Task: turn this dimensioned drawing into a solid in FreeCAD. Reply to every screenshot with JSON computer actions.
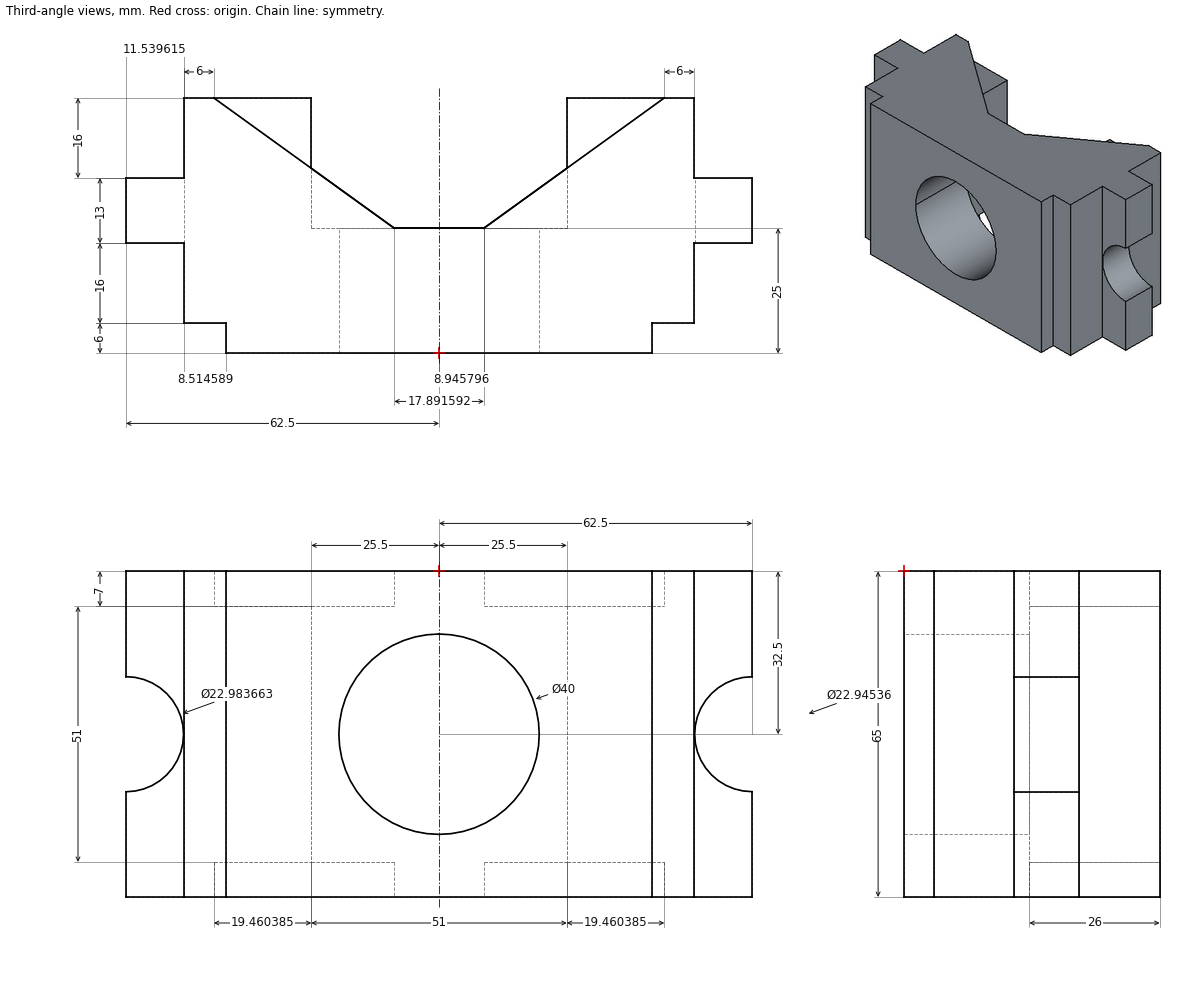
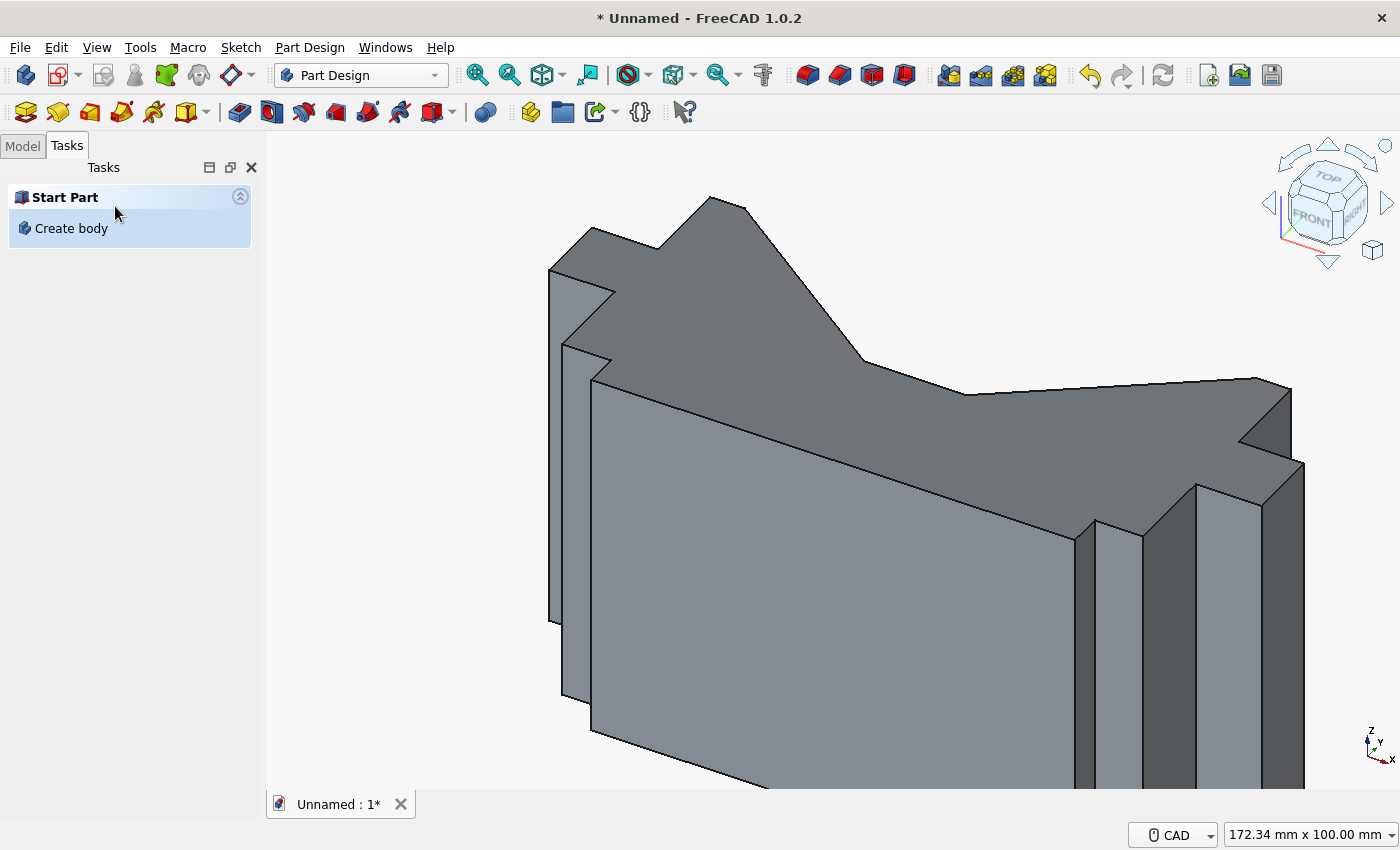
{"action": "left_click", "coordinate": [478, 76]}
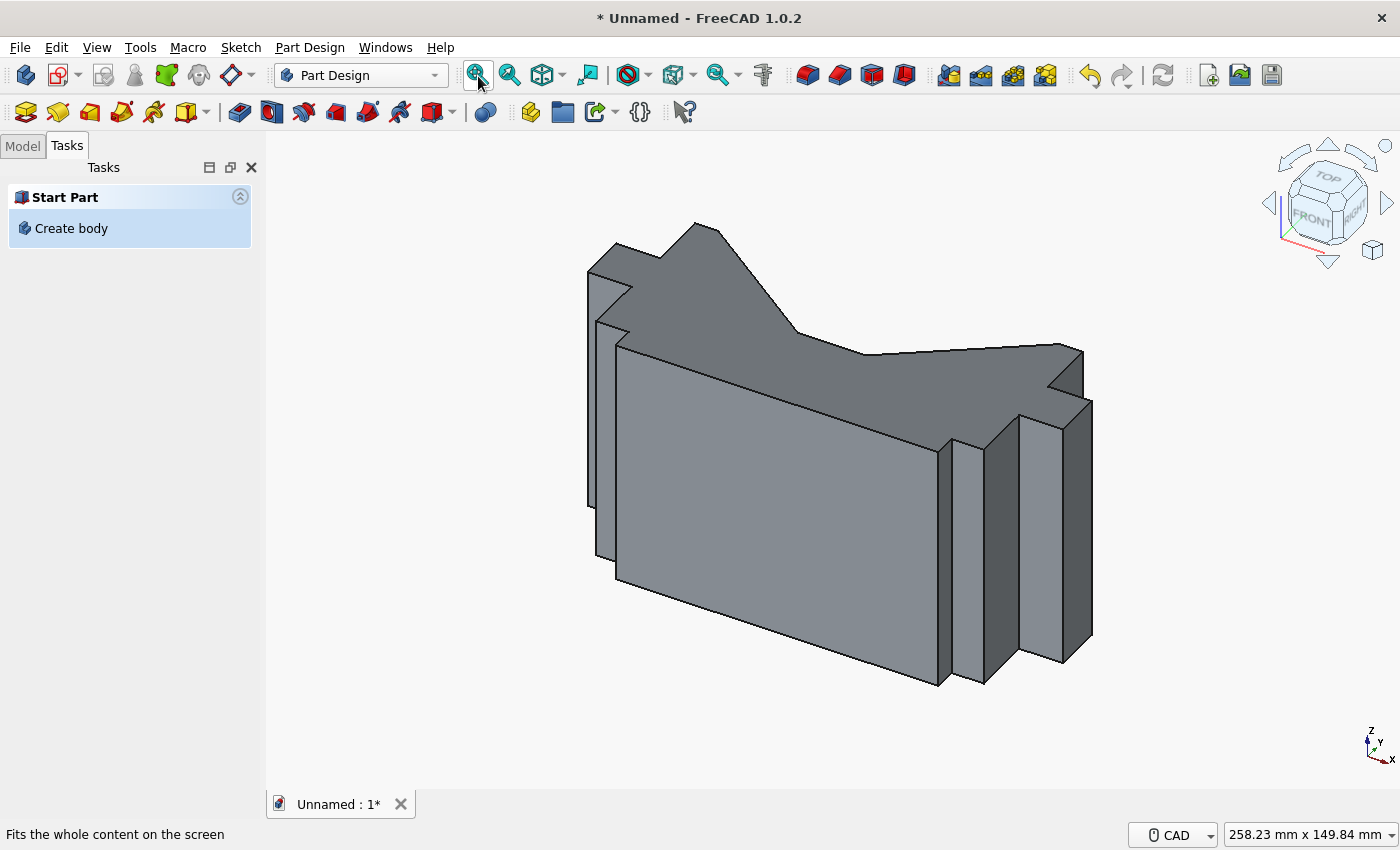
{"action": "key", "text": "4"}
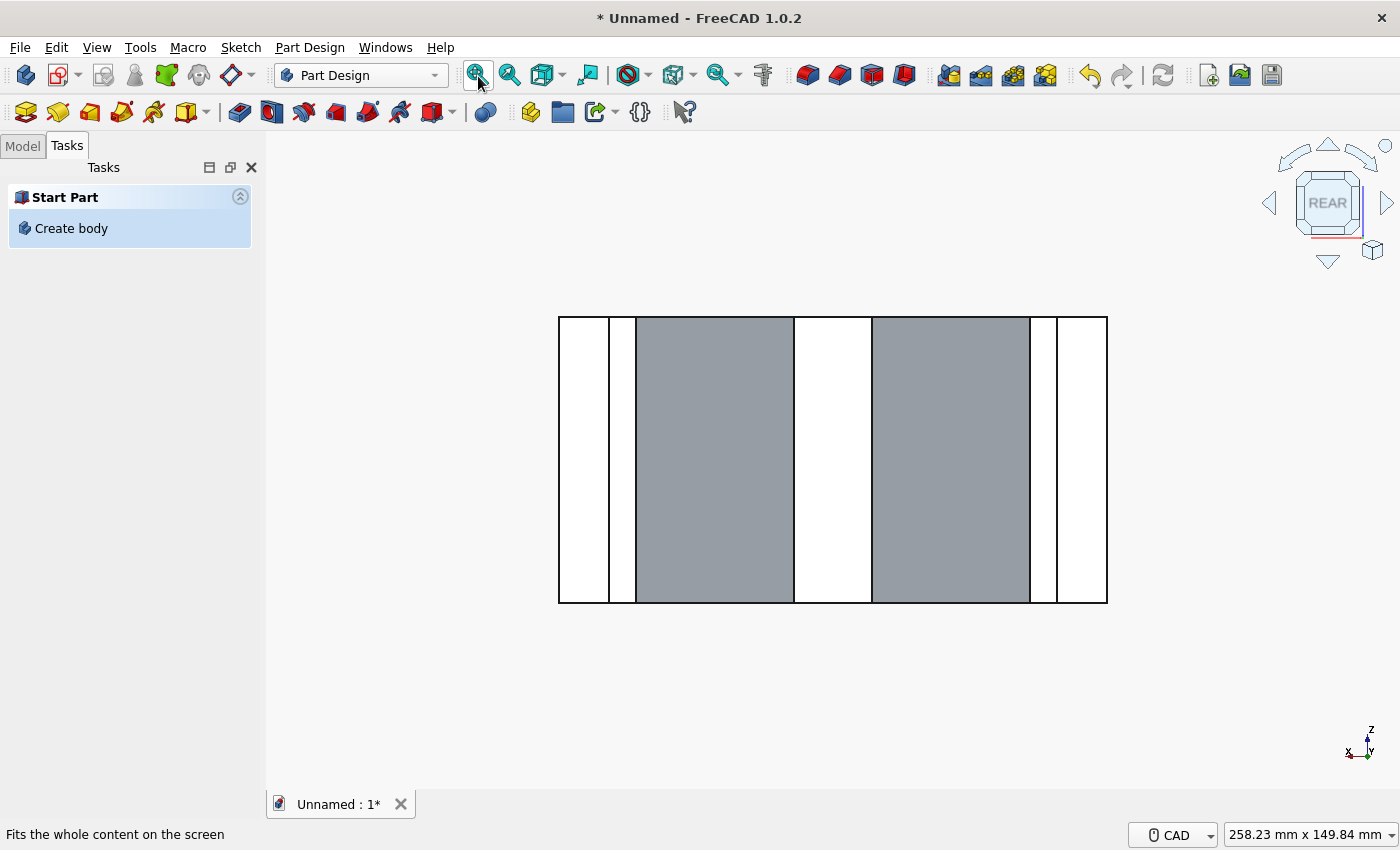
{"action": "left_click", "coordinate": [833, 377]}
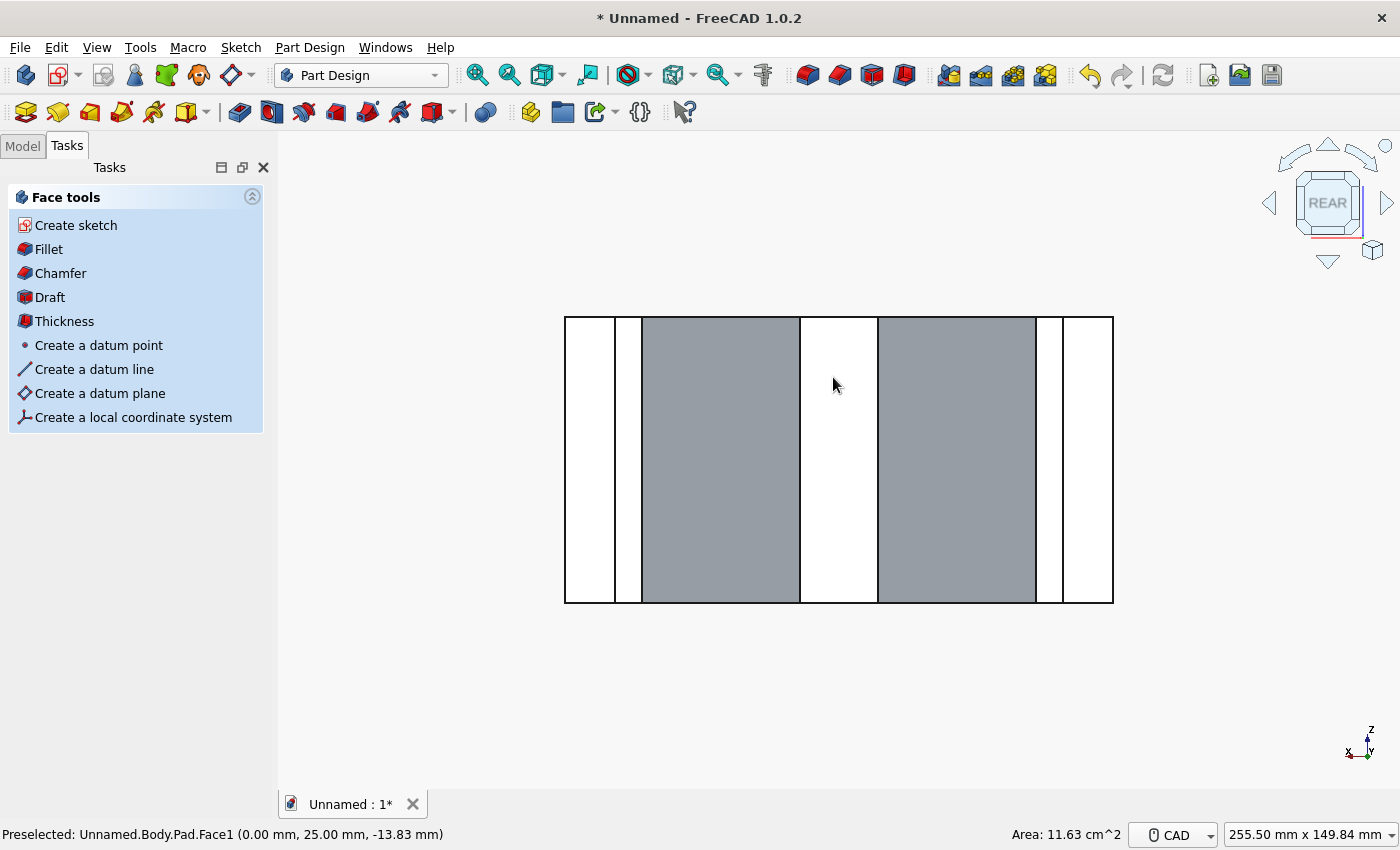
{"action": "left_click", "coordinate": [58, 76]}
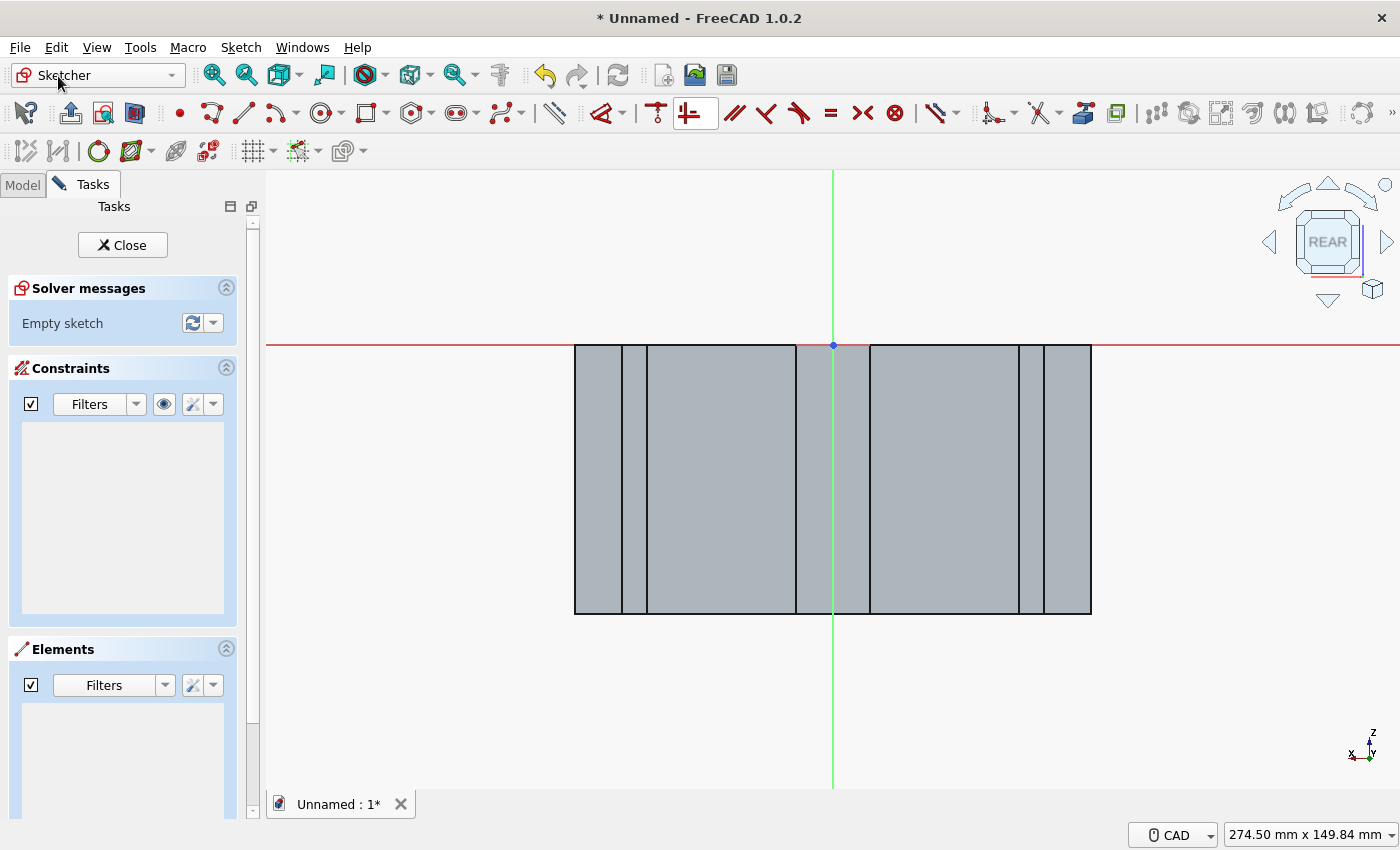
{"action": "scroll", "coordinate": [916, 447], "scroll_direction": "up", "scroll_amount": 3}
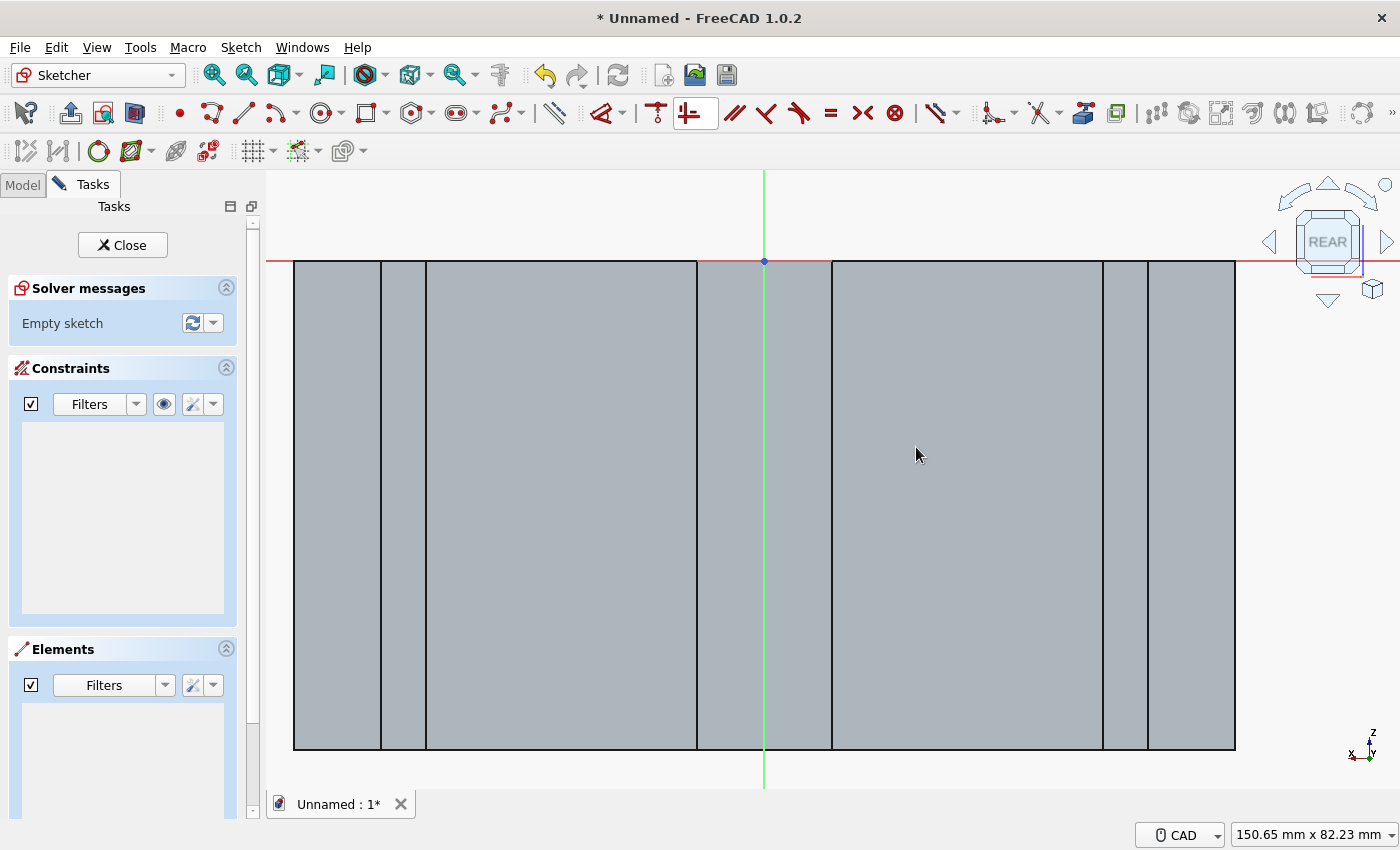
{"action": "left_click", "coordinate": [366, 114]}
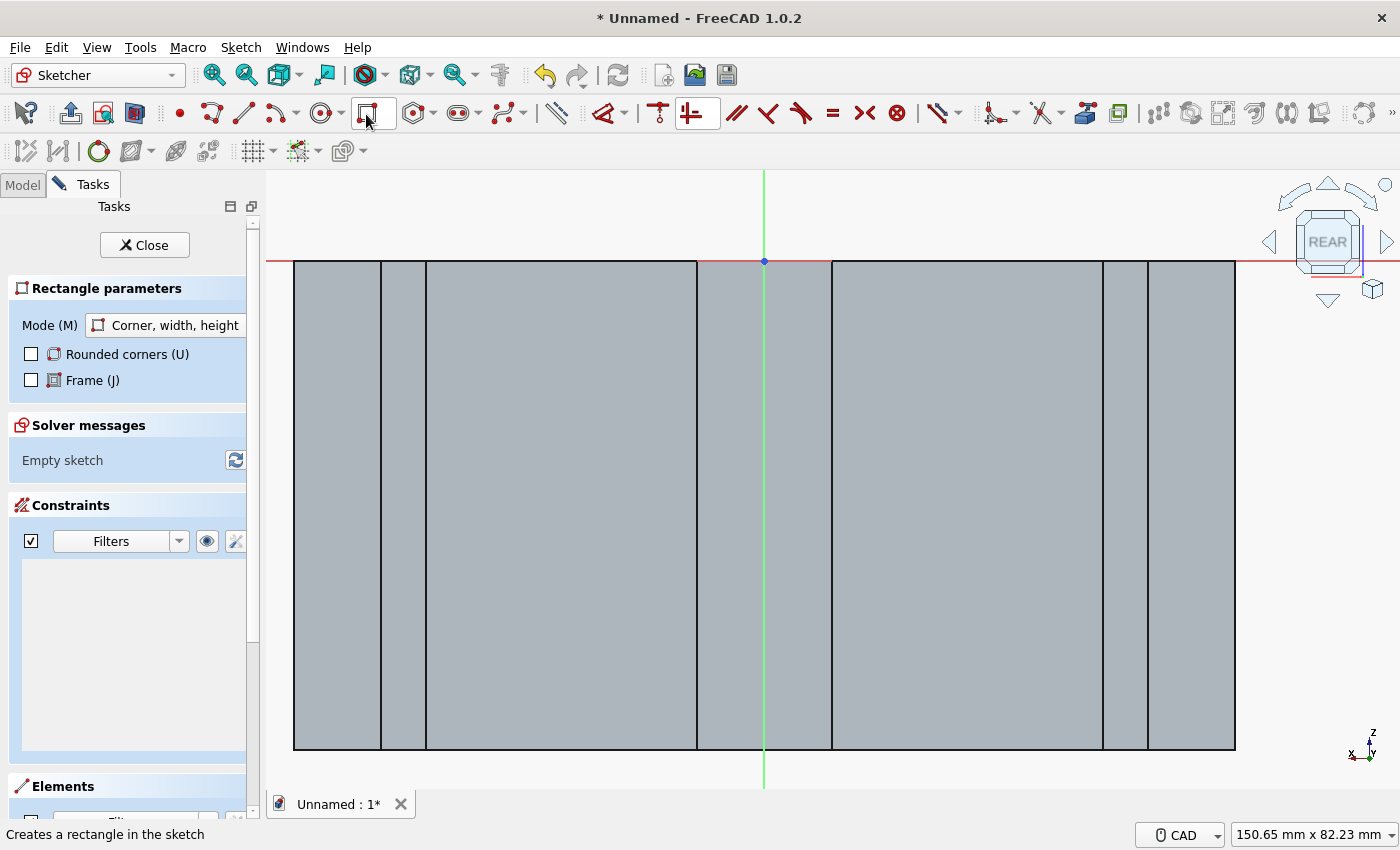
{"action": "left_click", "coordinate": [956, 314]}
{"action": "mouse_move", "coordinate": [1103, 698]}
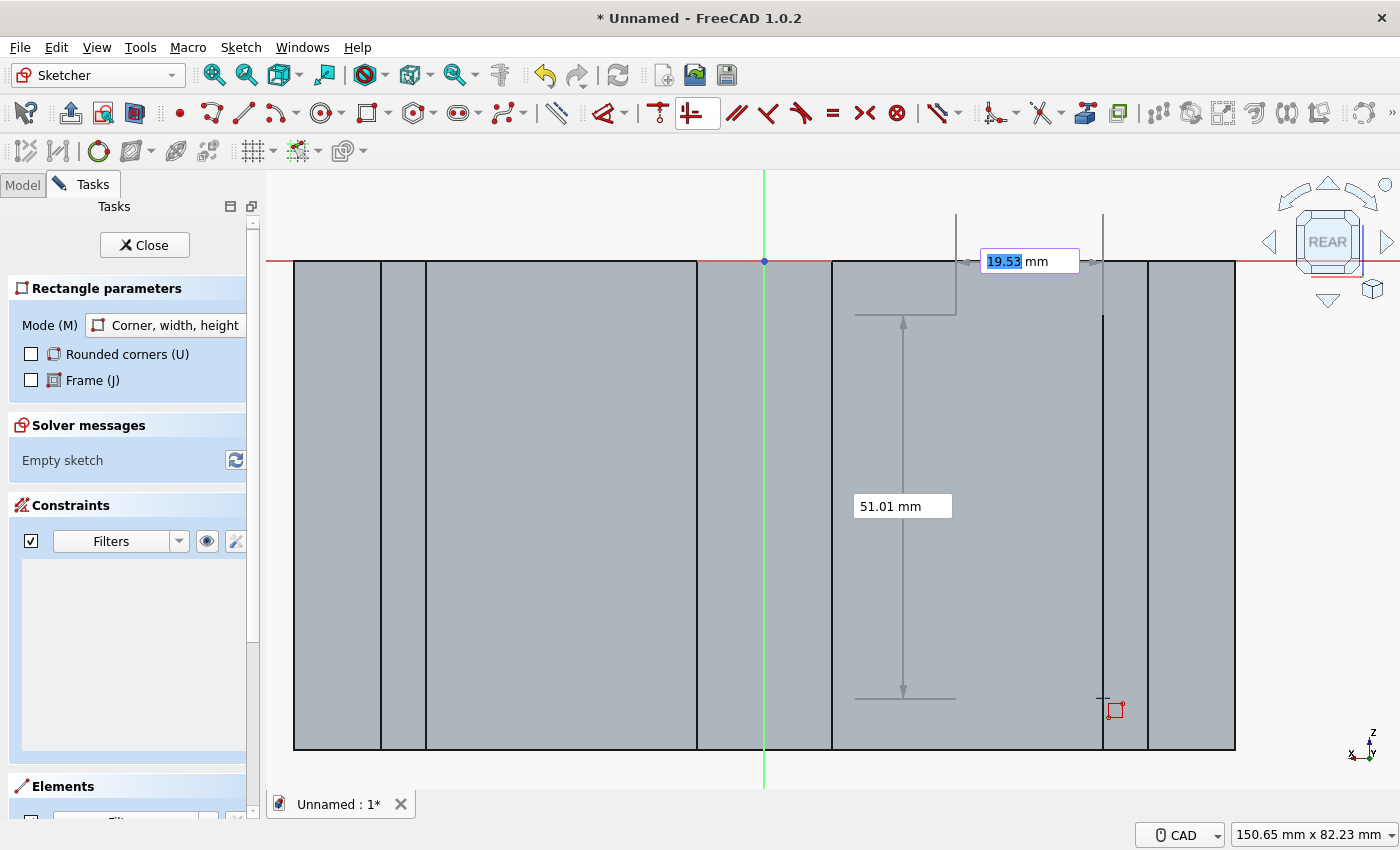
{"action": "type", "text": "19.460385"}
{"action": "key", "text": "Tab"}
{"action": "type", "text": "51"}
{"action": "key", "text": "Return"}